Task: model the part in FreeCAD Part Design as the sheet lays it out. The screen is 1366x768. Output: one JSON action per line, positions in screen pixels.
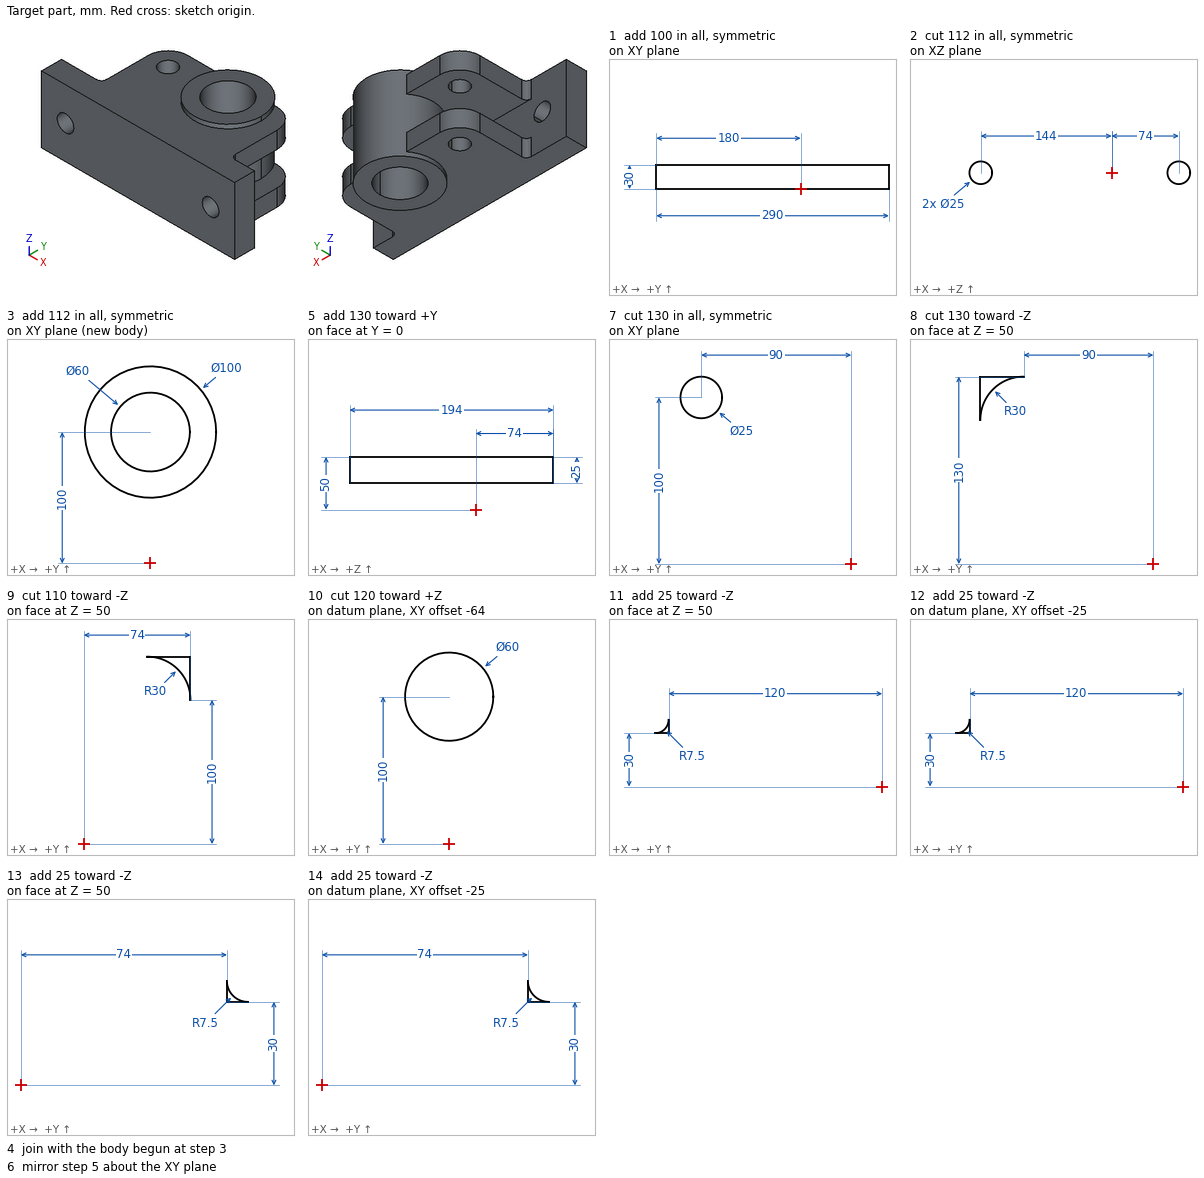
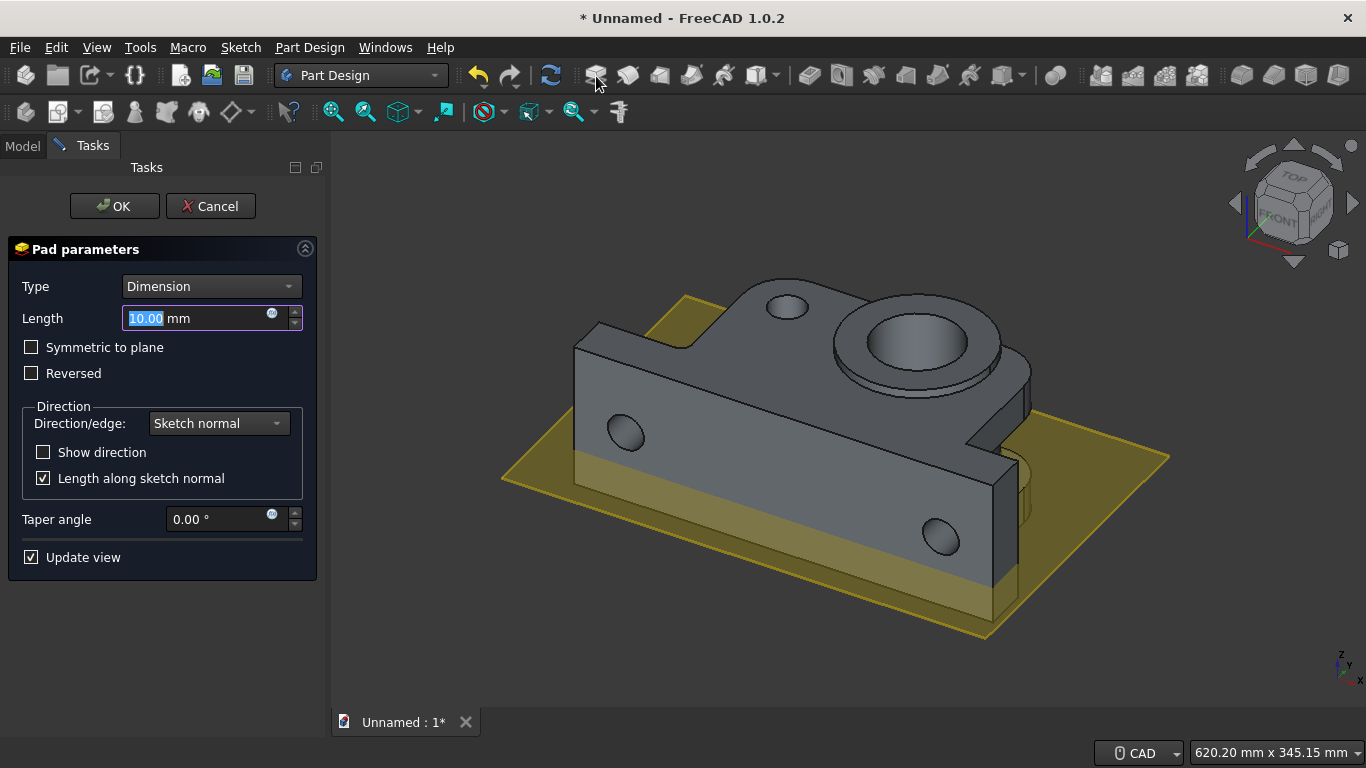
{"action": "type", "text": "25"}
{"action": "key", "text": "Tab"}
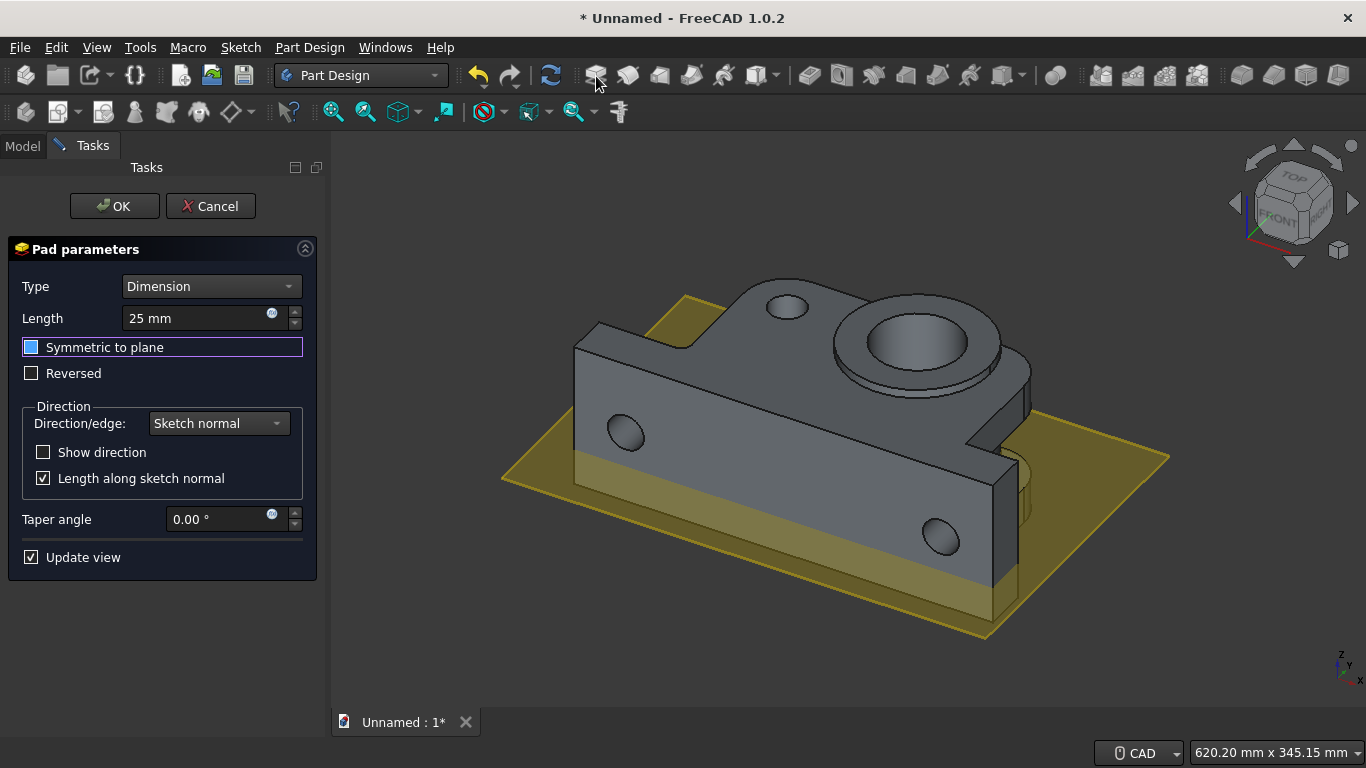
{"action": "left_click", "coordinate": [30, 373]}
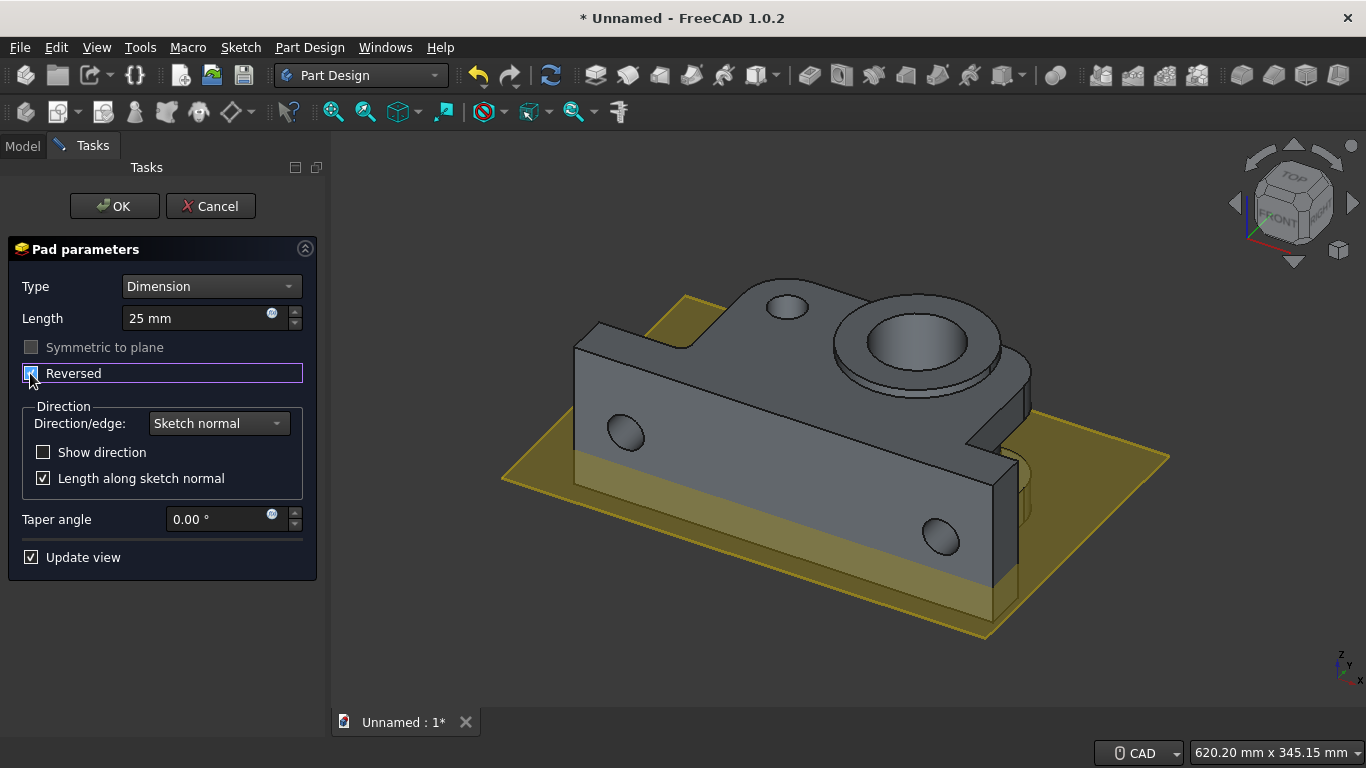
{"action": "left_click", "coordinate": [115, 206]}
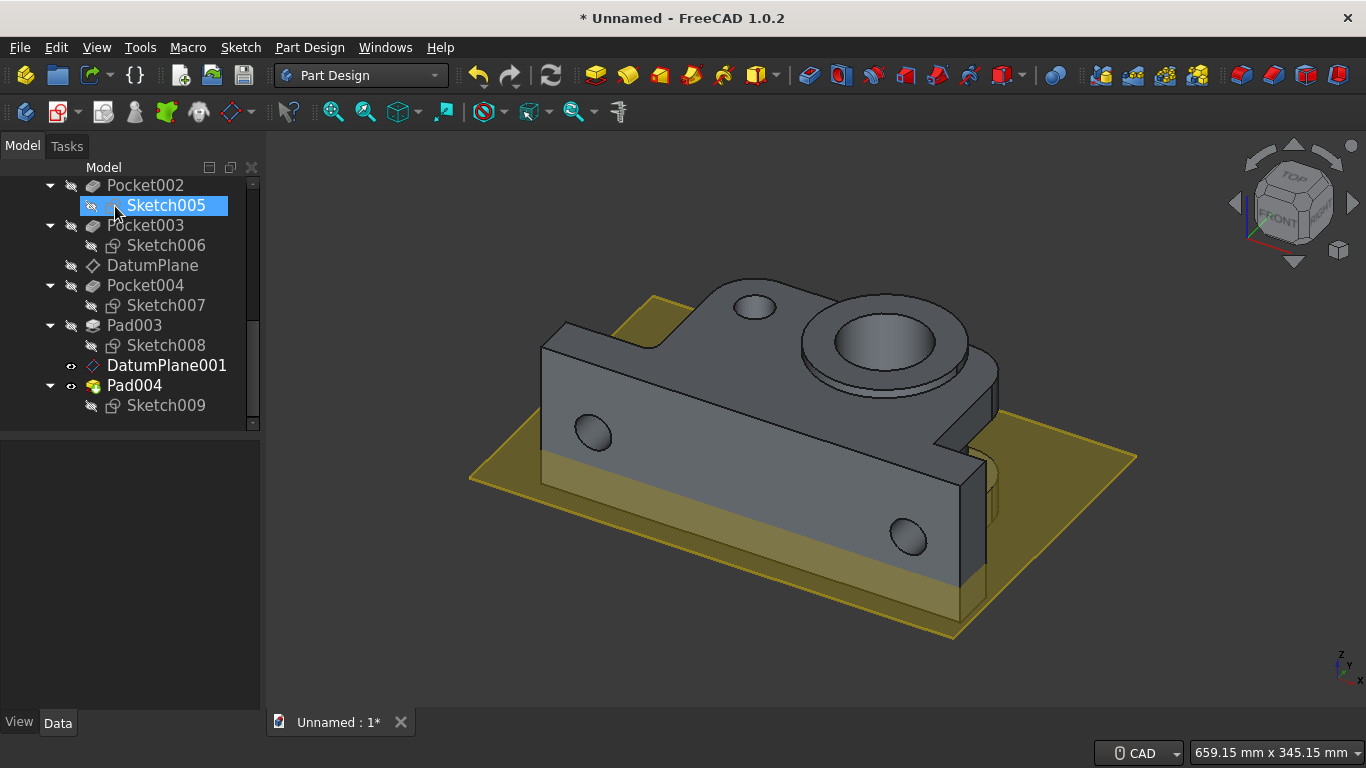
{"action": "left_click", "coordinate": [116, 366]}
{"action": "key", "text": "space"}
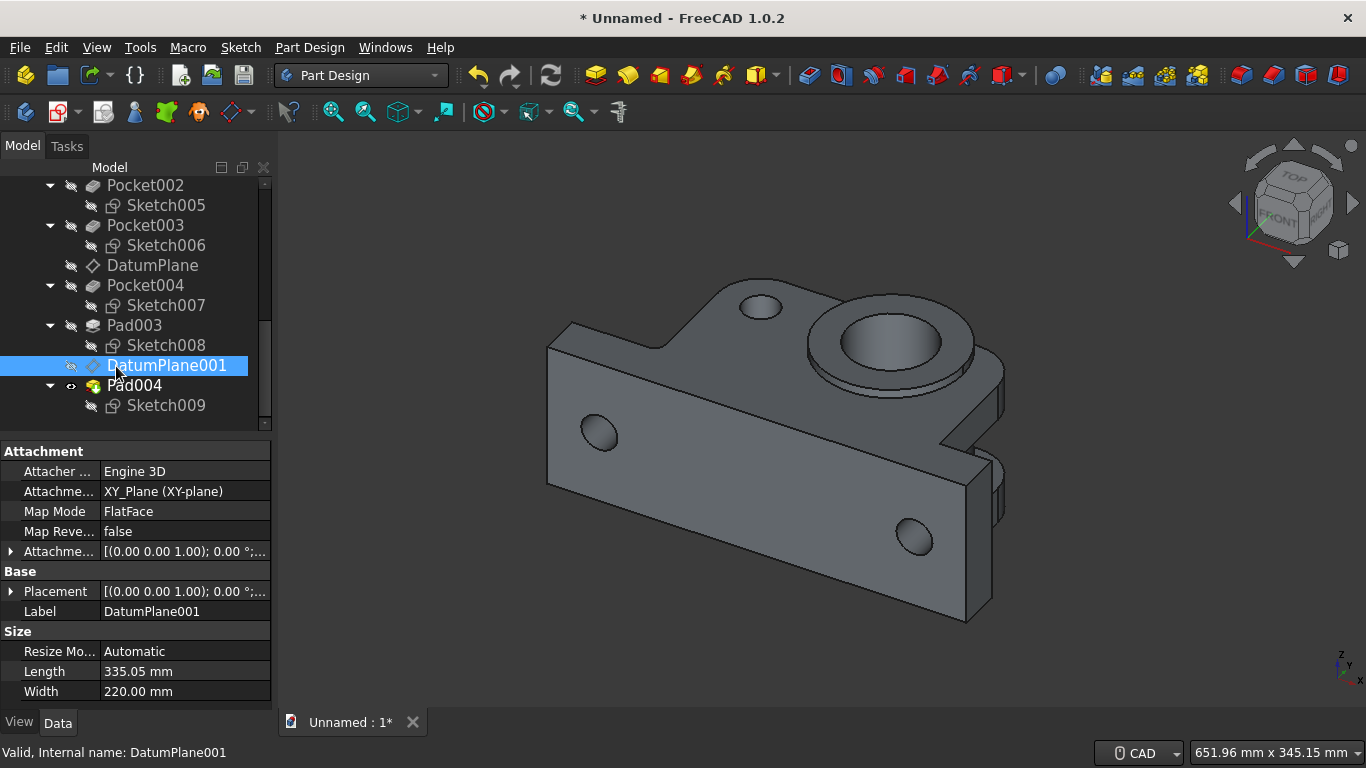
{"action": "left_click", "coordinate": [736, 357]}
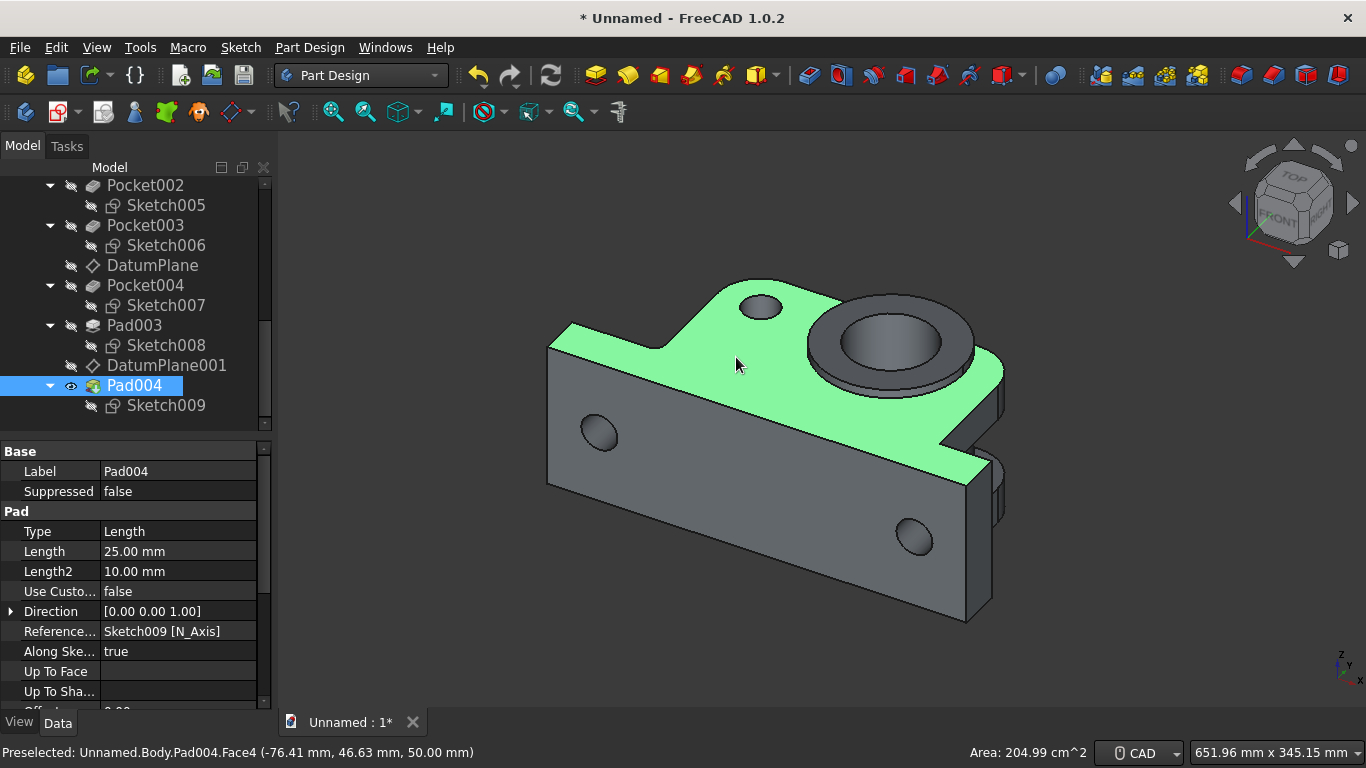
{"action": "left_click", "coordinate": [58, 112]}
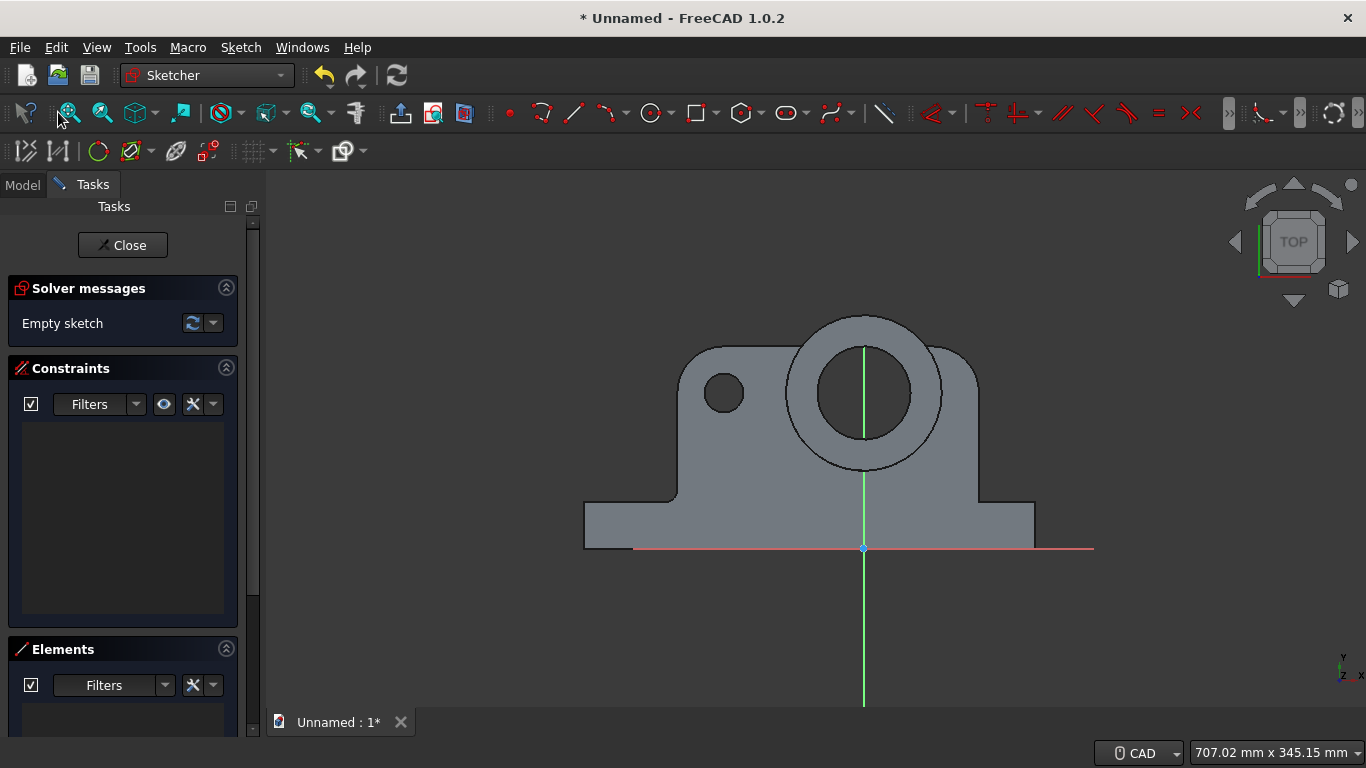
{"action": "scroll", "coordinate": [997, 499], "scroll_direction": "up", "scroll_amount": 15}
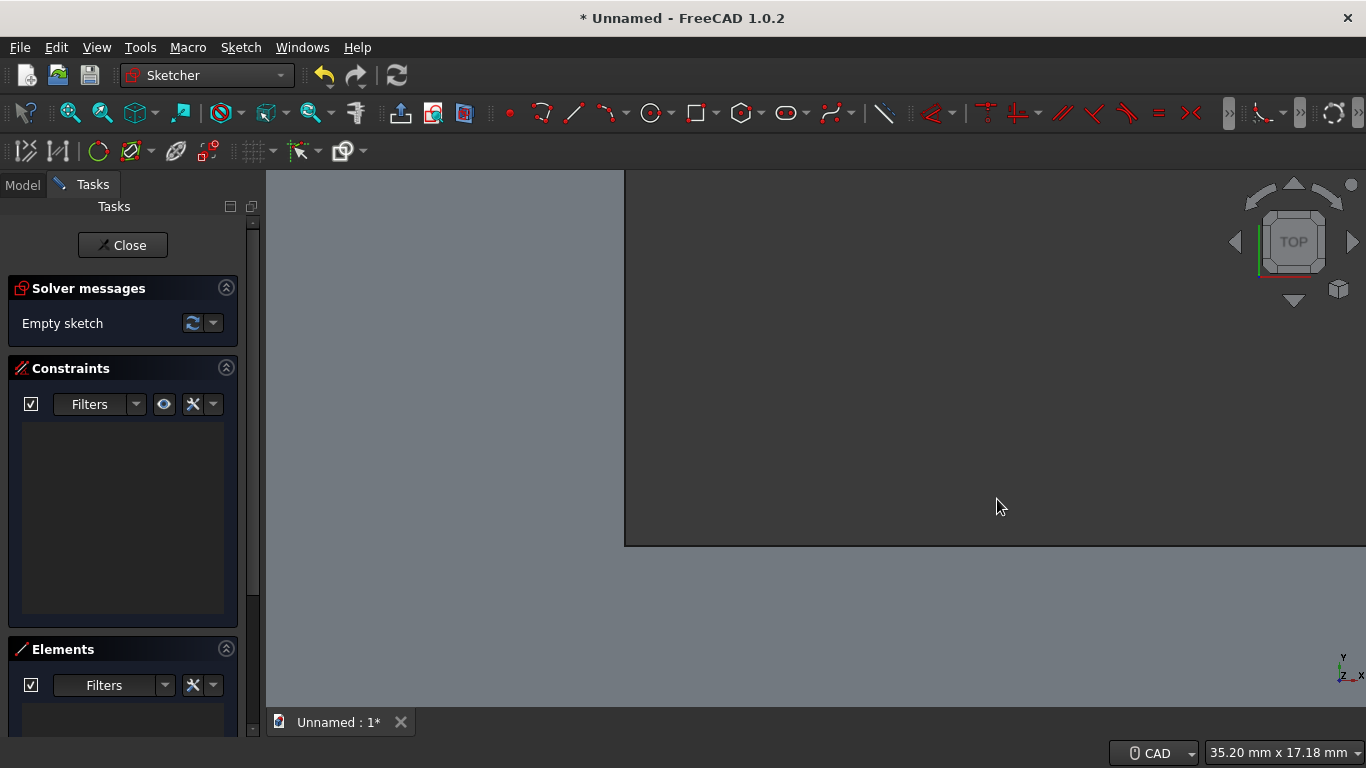
{"action": "scroll", "coordinate": [731, 408], "scroll_direction": "up", "scroll_amount": 2}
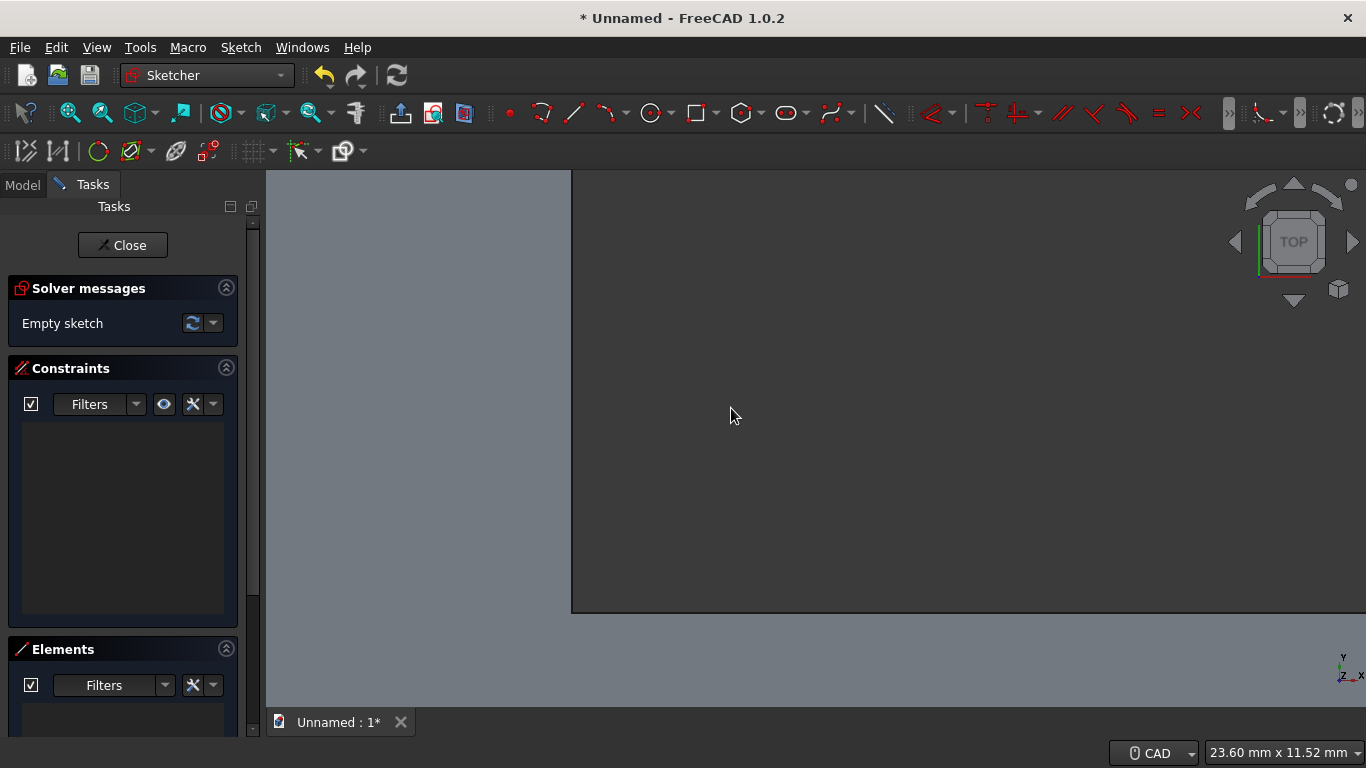
{"action": "left_click", "coordinate": [542, 114]}